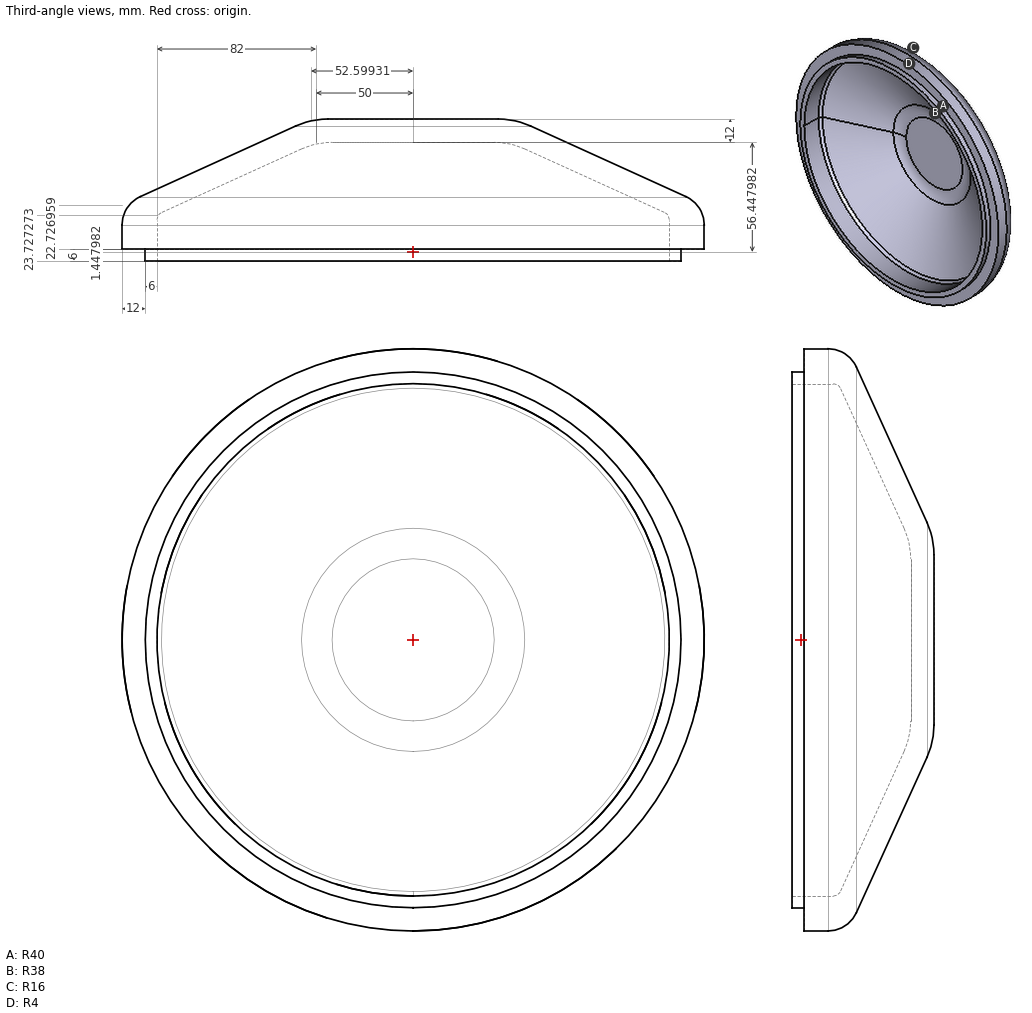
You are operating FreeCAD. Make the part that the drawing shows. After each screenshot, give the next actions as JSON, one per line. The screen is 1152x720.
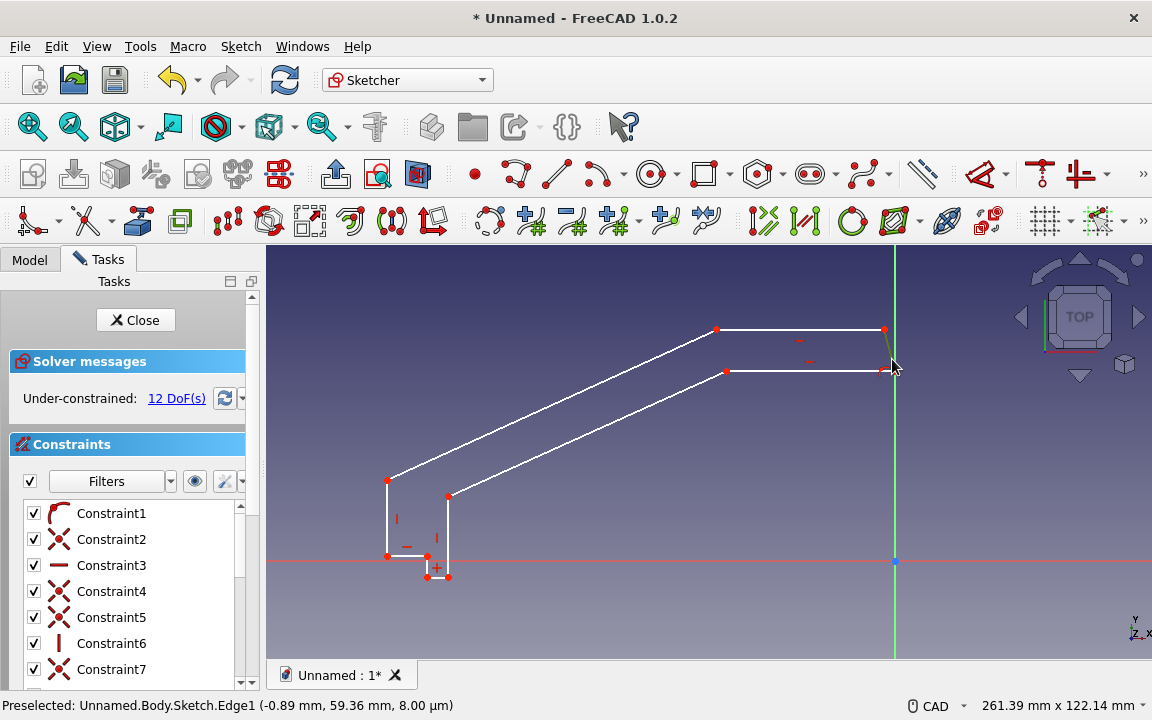
{"action": "key", "text": "v"}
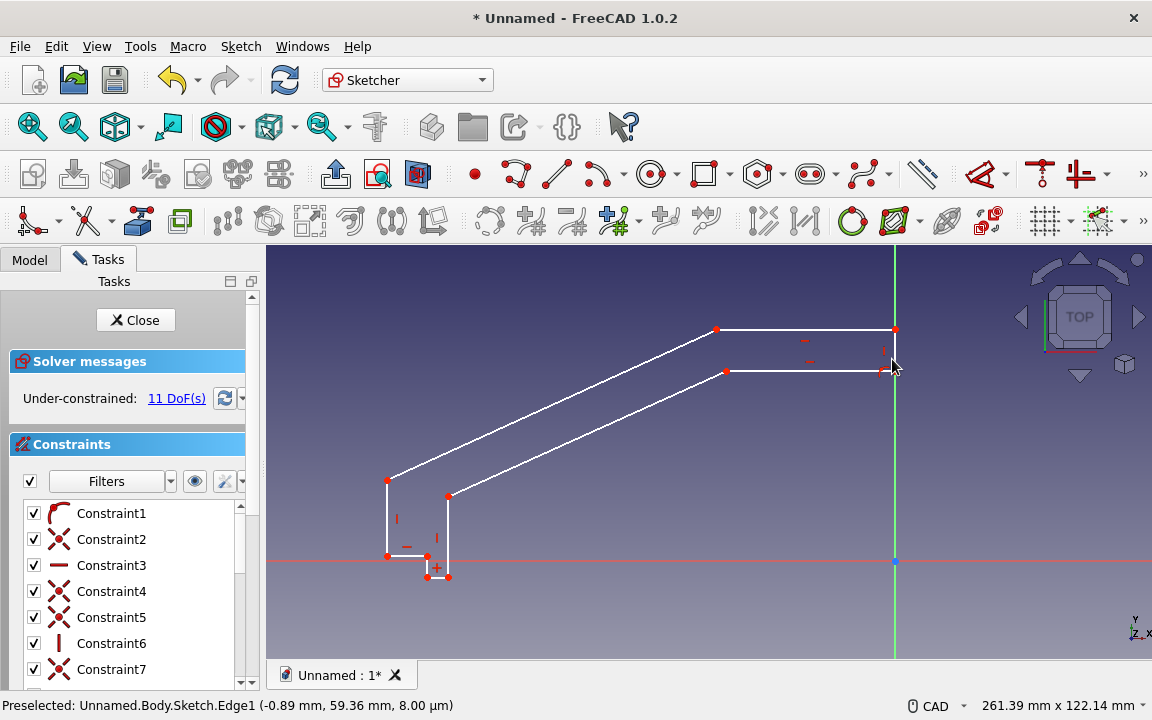
{"action": "key", "text": "d"}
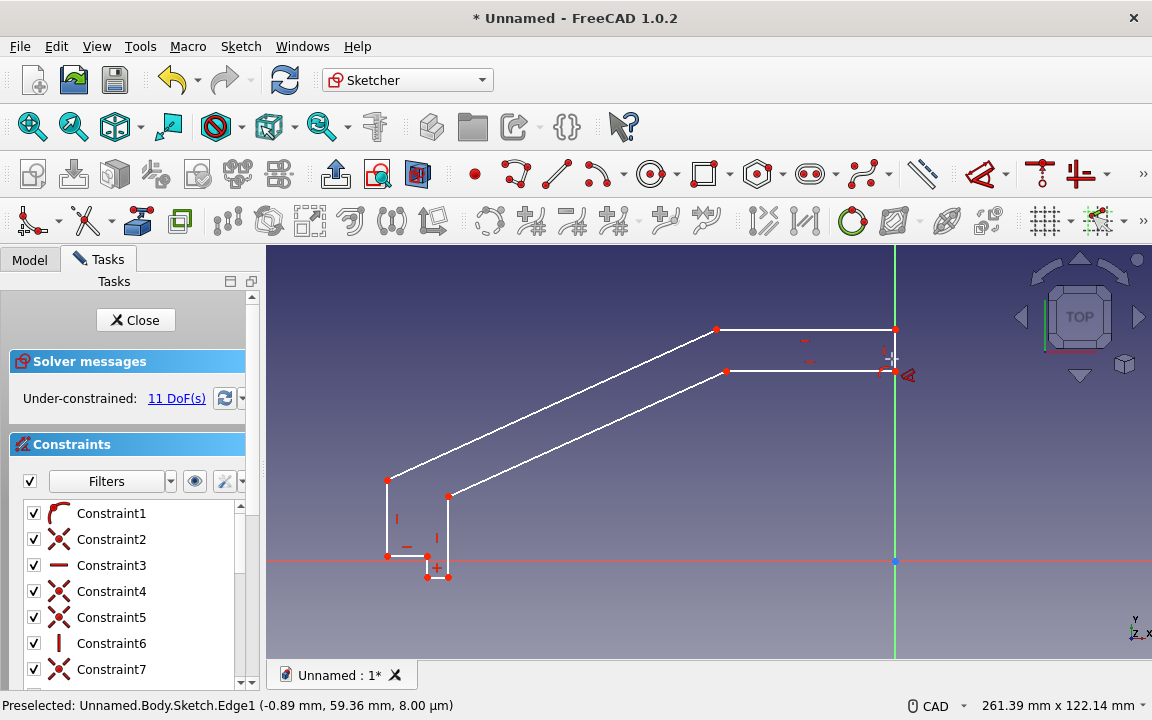
{"action": "scroll", "coordinate": [427, 565], "scroll_direction": "up", "scroll_amount": 4}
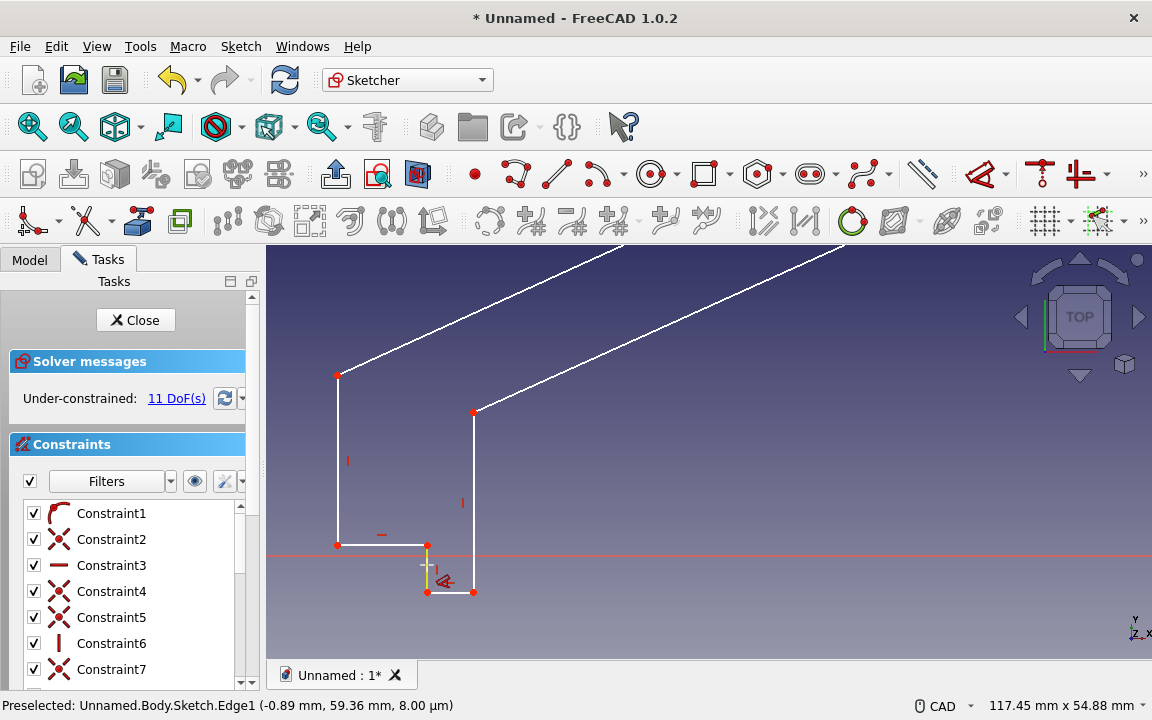
{"action": "left_click", "coordinate": [427, 564]}
{"action": "left_click", "coordinate": [393, 569]}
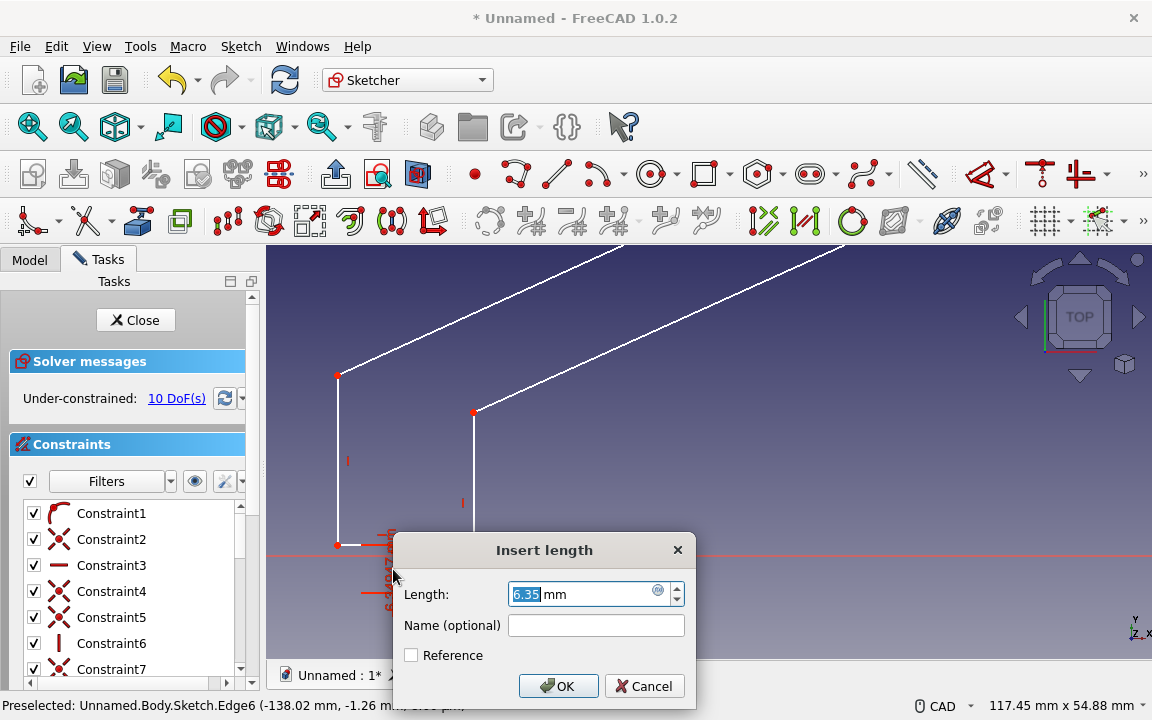
{"action": "type", "text": "6"}
{"action": "key", "text": "Return"}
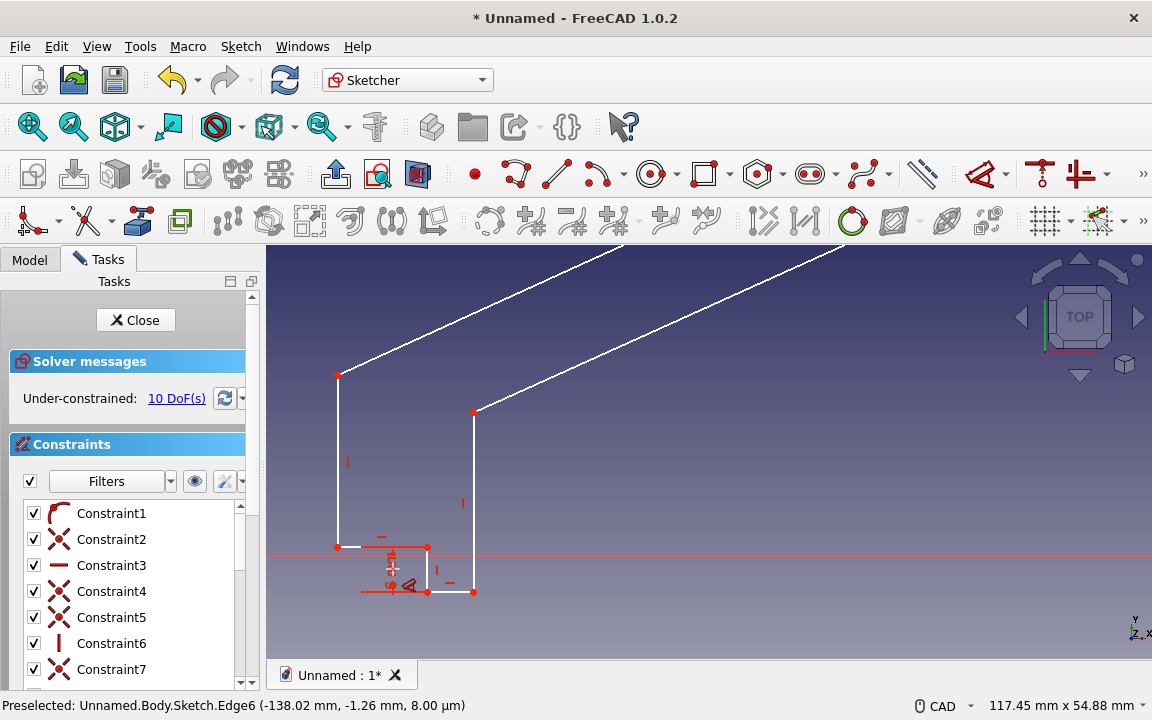
{"action": "left_click", "coordinate": [441, 592]}
{"action": "left_click", "coordinate": [450, 626]}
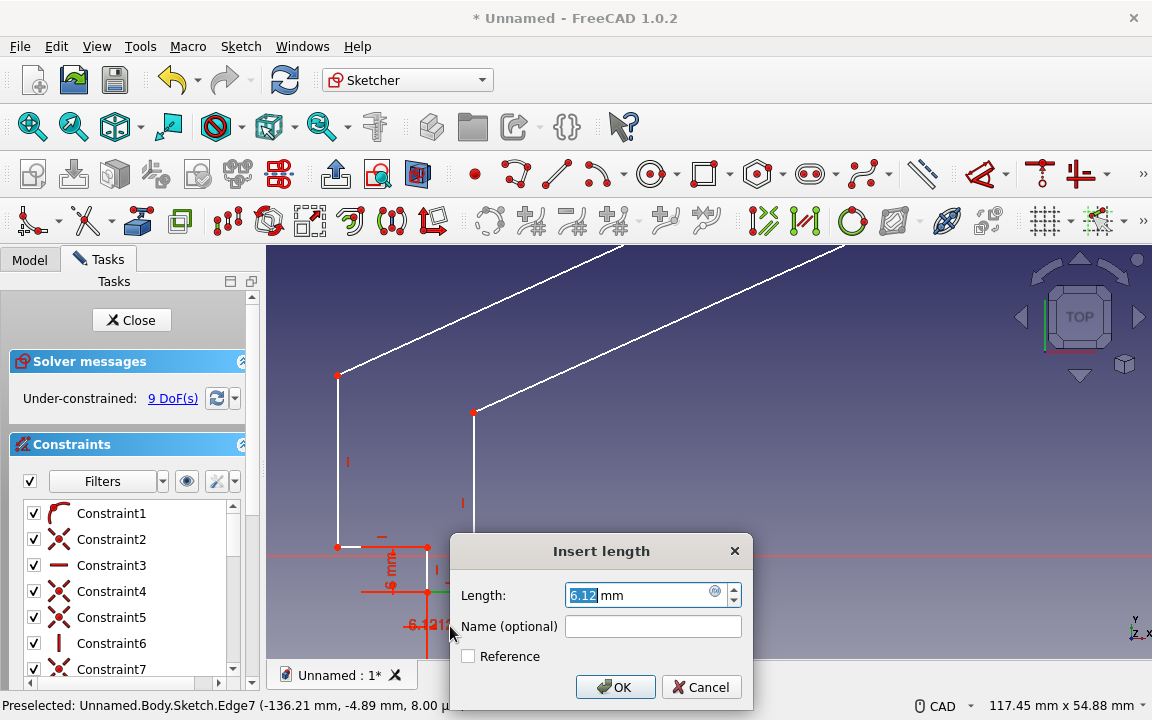
{"action": "type", "text": "6"}
{"action": "key", "text": "Return"}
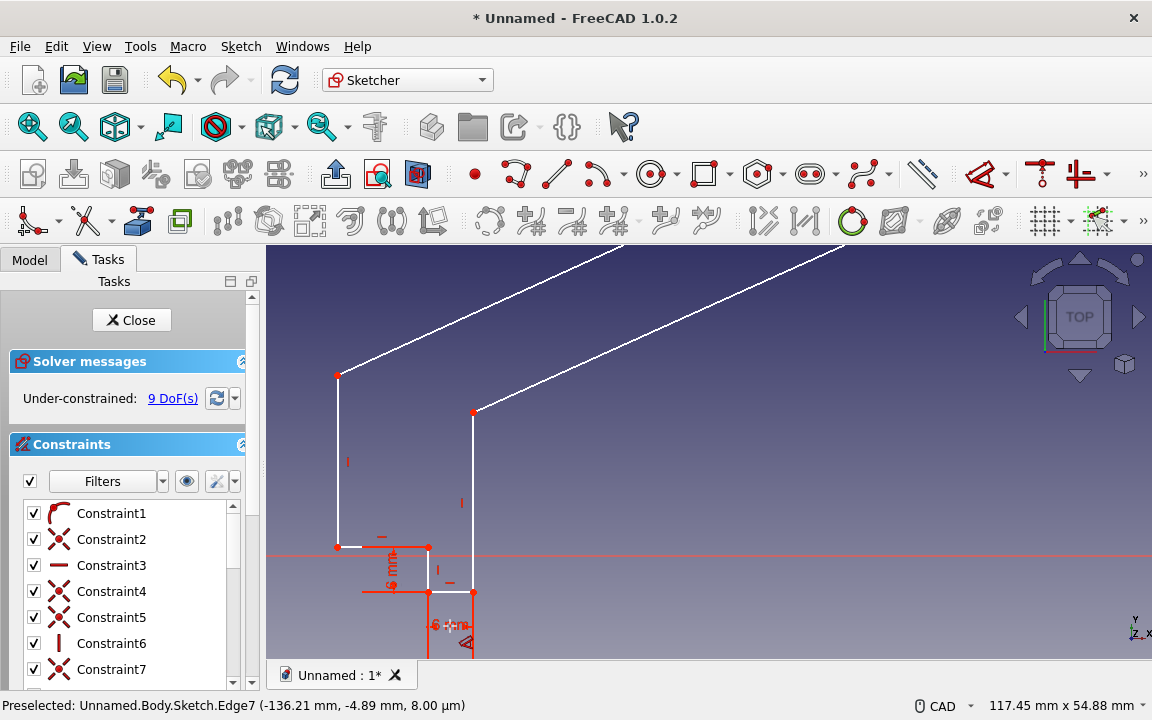
{"action": "scroll", "coordinate": [427, 564], "scroll_direction": "down", "scroll_amount": 4}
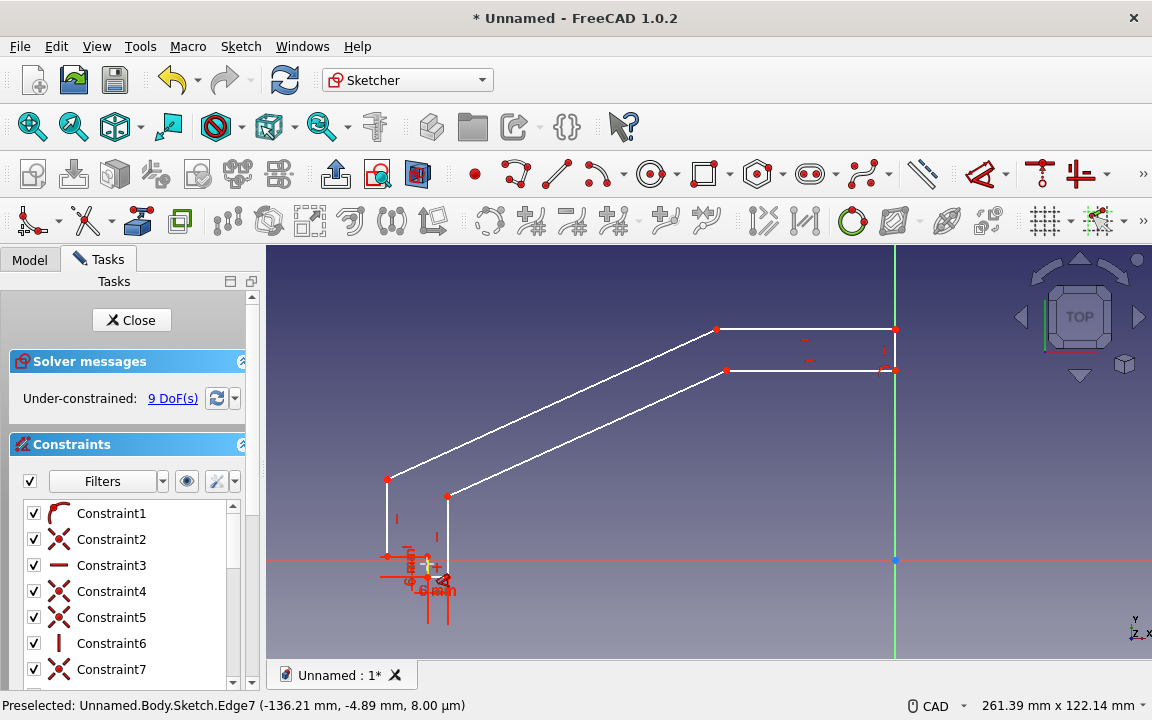
{"action": "left_click", "coordinate": [895, 358]}
{"action": "left_click", "coordinate": [929, 350]}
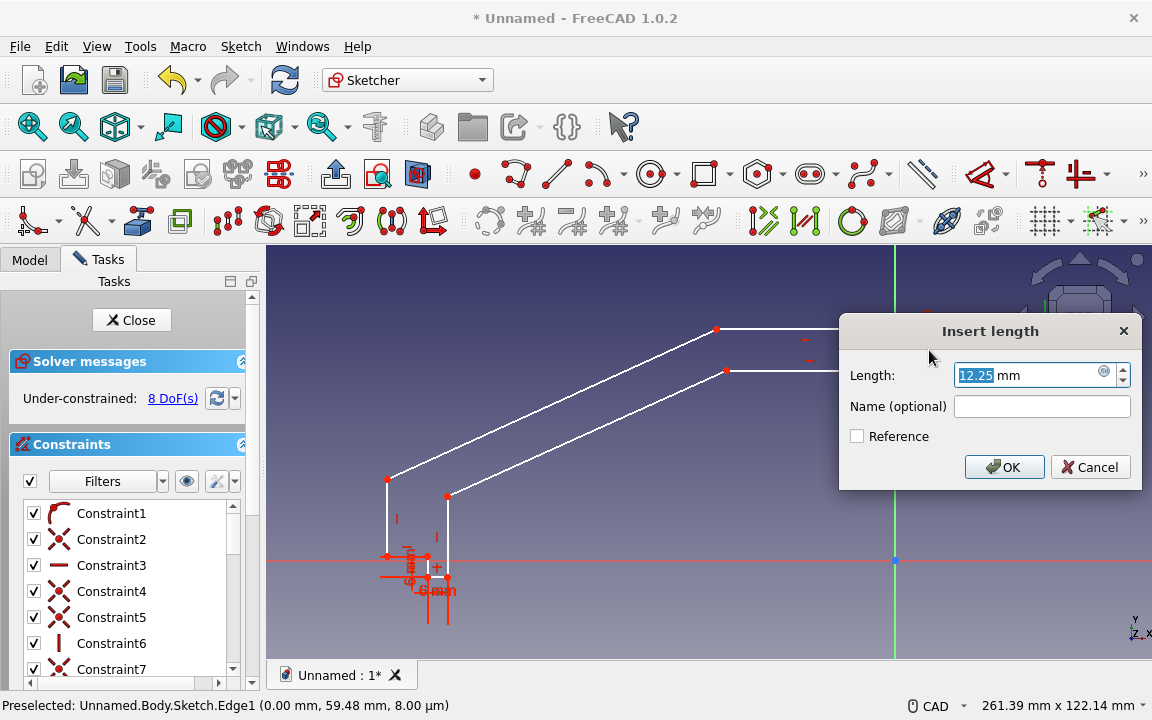
{"action": "type", "text": "12"}
{"action": "key", "text": "Return"}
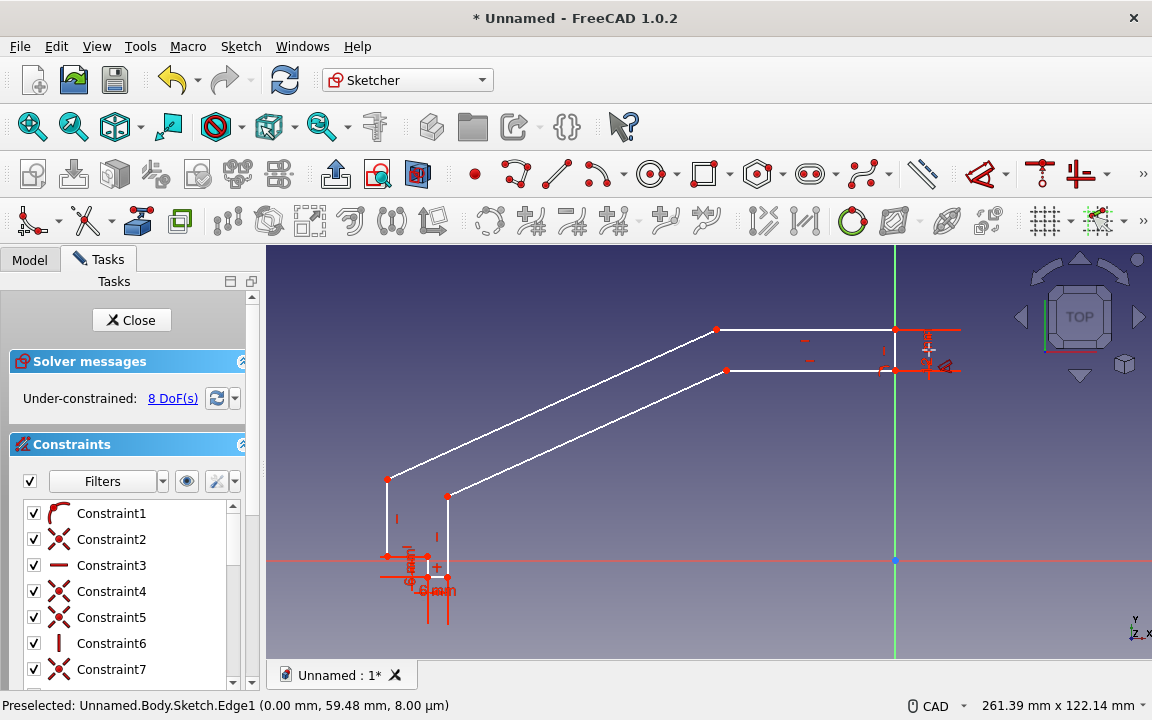
{"action": "left_click", "coordinate": [399, 557]}
{"action": "left_click", "coordinate": [407, 523]}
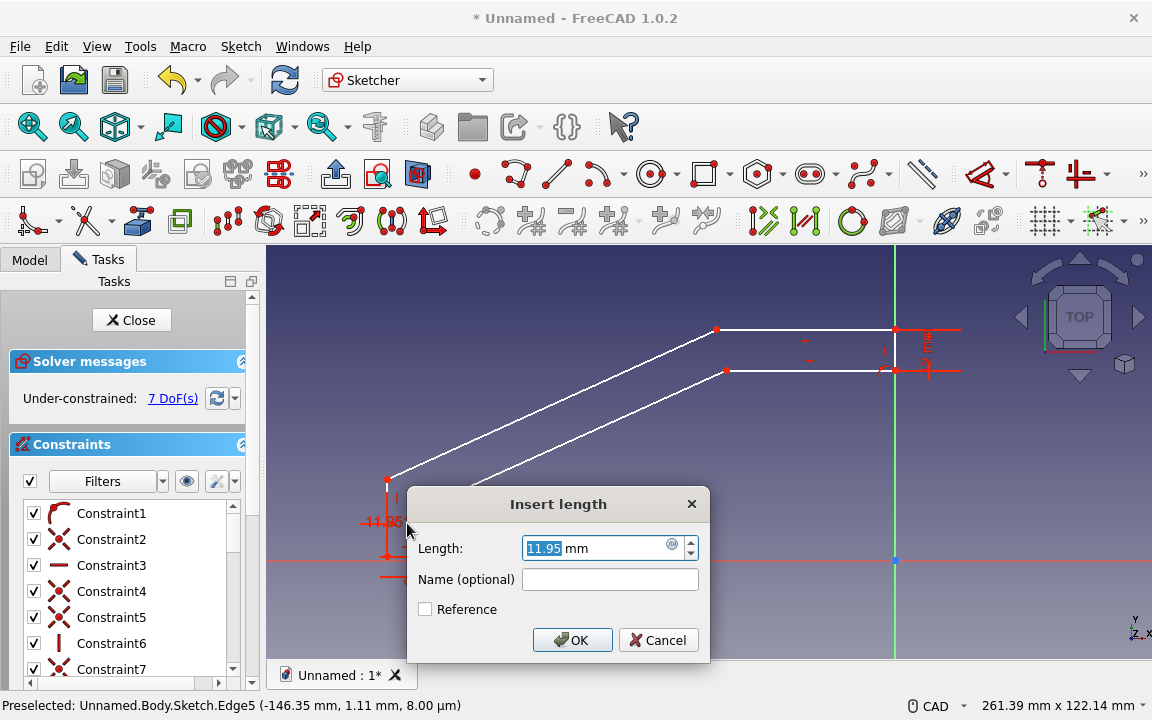
{"action": "type", "text": "12"}
{"action": "key", "text": "Return"}